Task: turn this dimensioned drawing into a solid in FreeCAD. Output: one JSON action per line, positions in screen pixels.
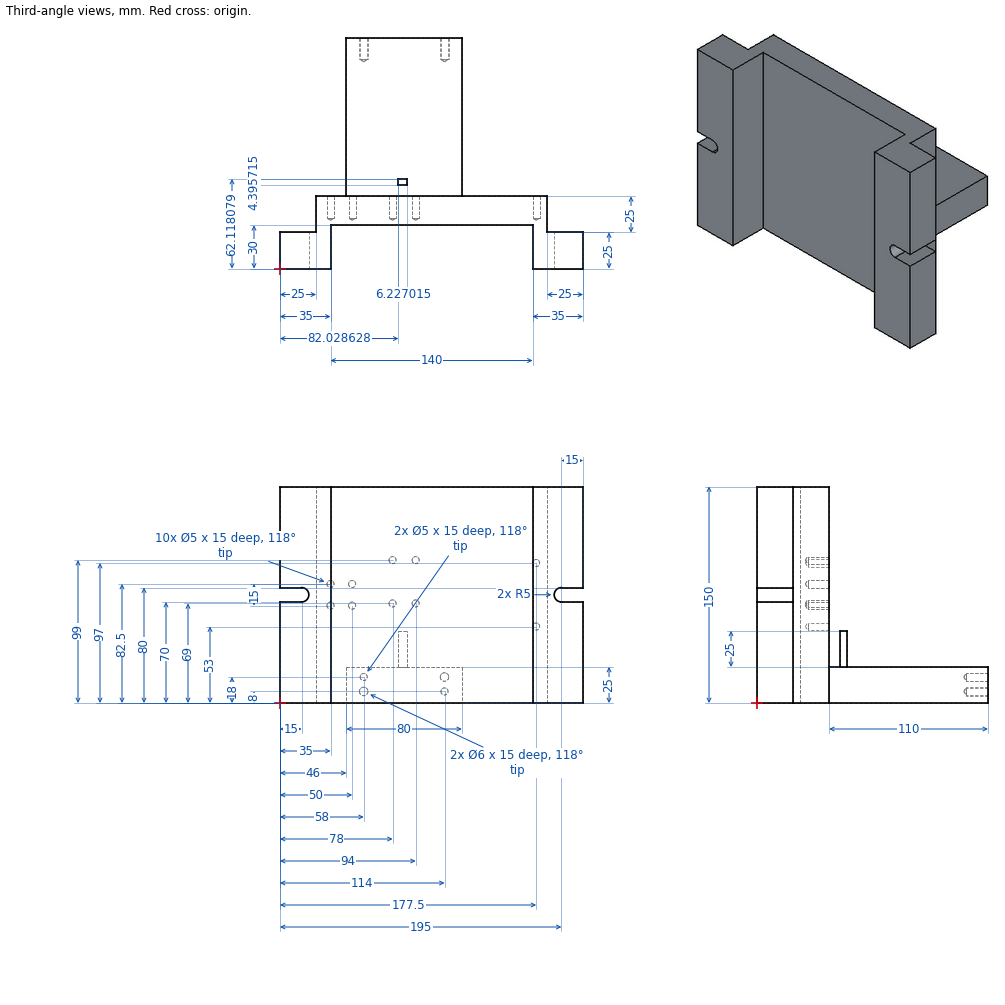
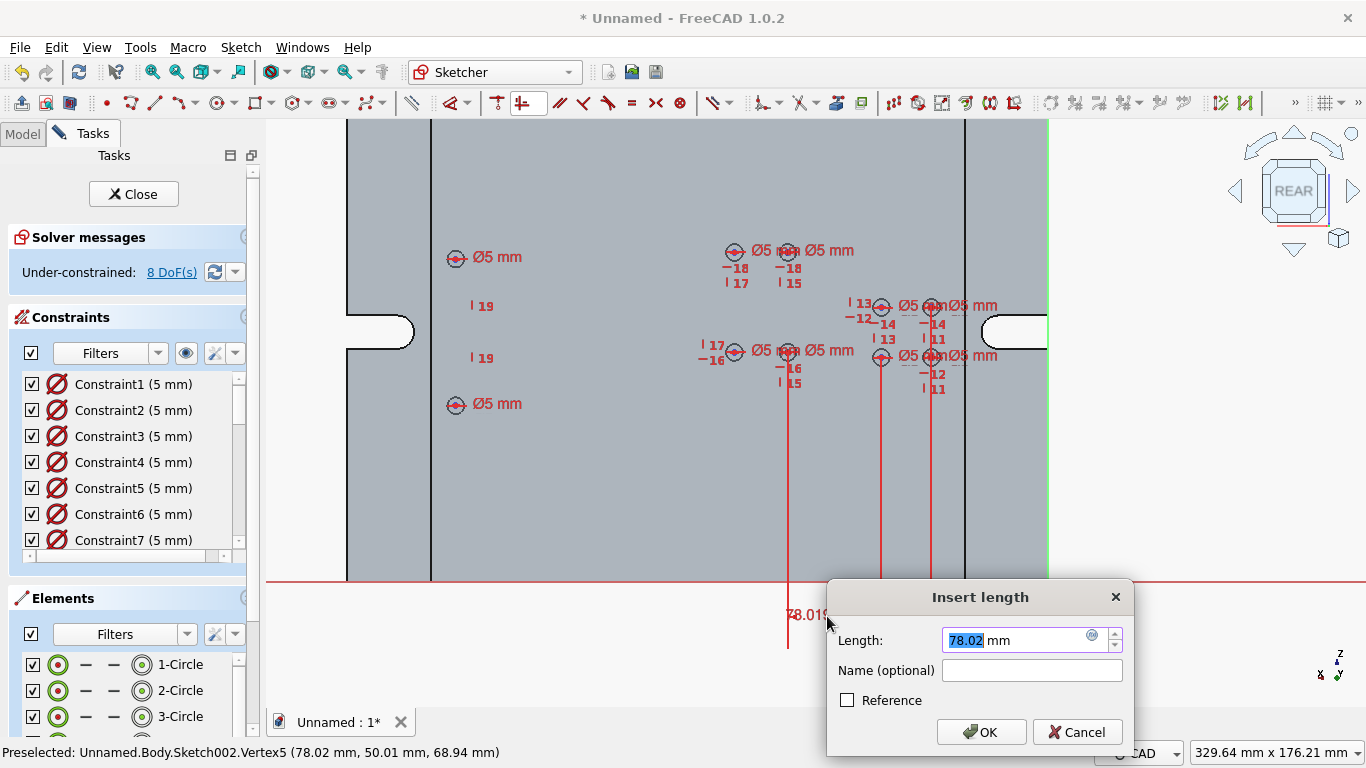
{"action": "type", "text": "78"}
{"action": "key", "text": "Return"}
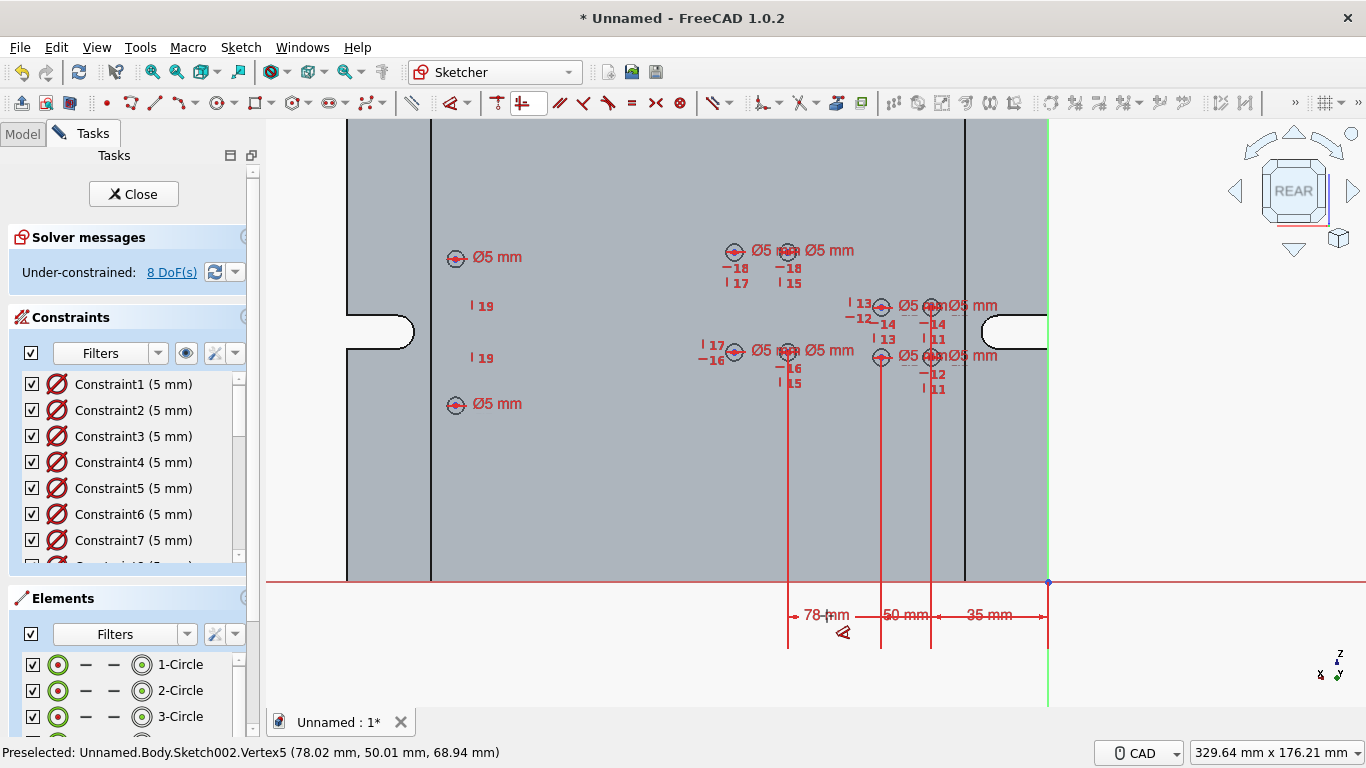
{"action": "left_click", "coordinate": [788, 352]}
{"action": "left_click", "coordinate": [1082, 467]}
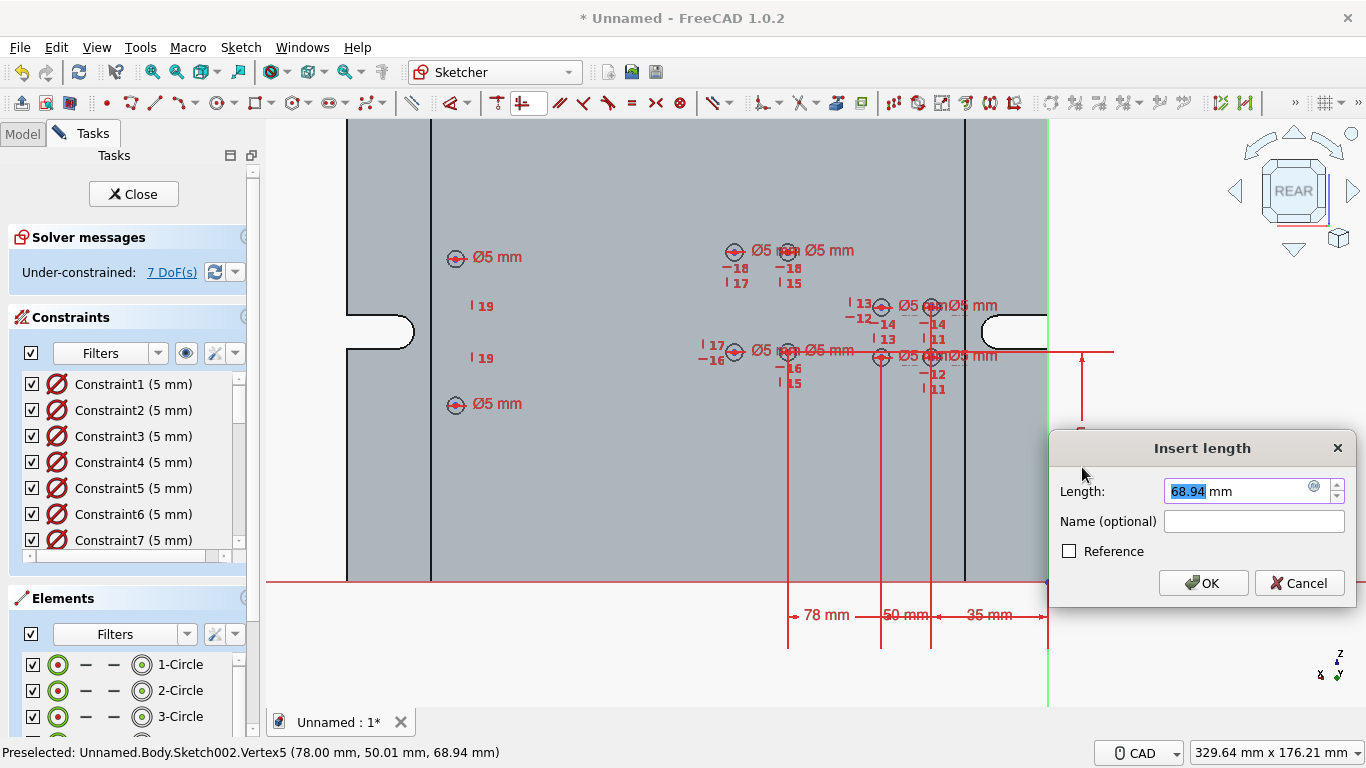
{"action": "type", "text": "69"}
{"action": "key", "text": "Return"}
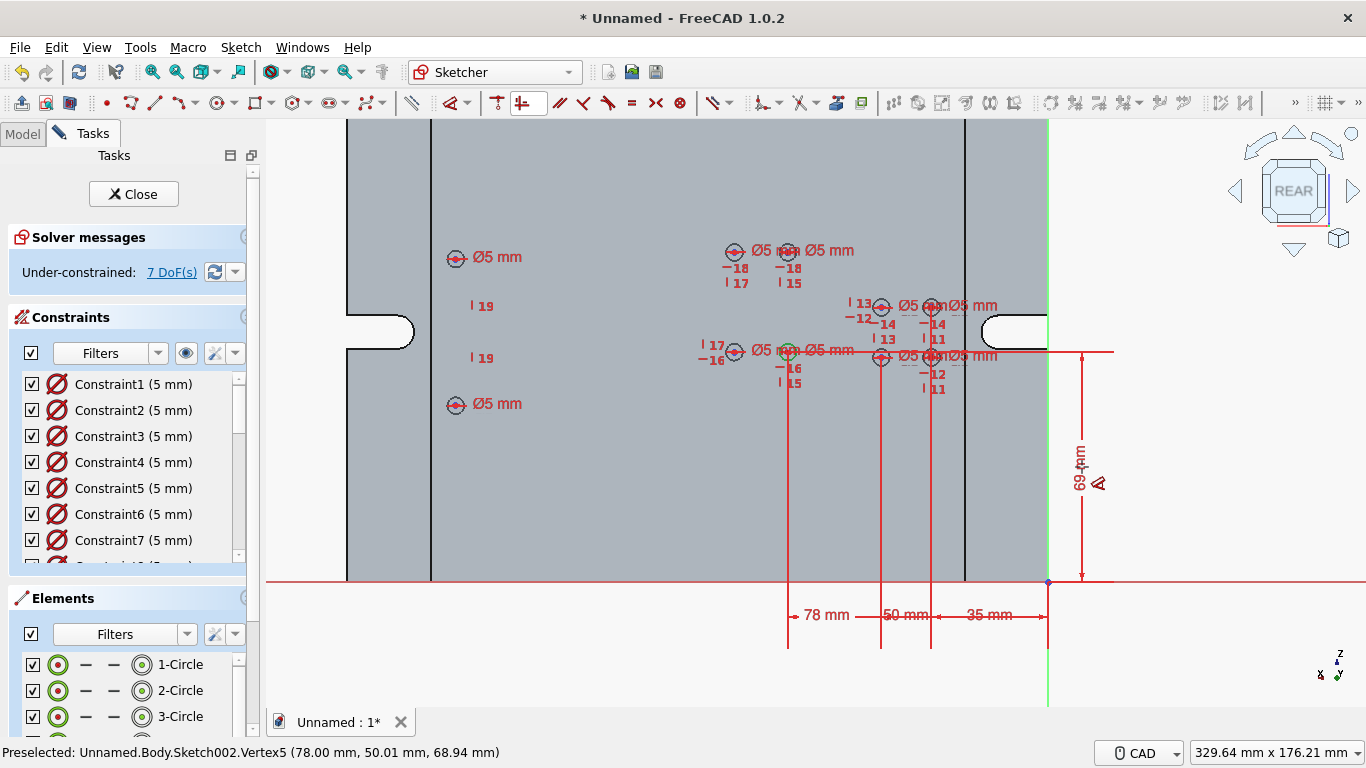
{"action": "left_click", "coordinate": [788, 252]}
{"action": "left_click", "coordinate": [1082, 417]}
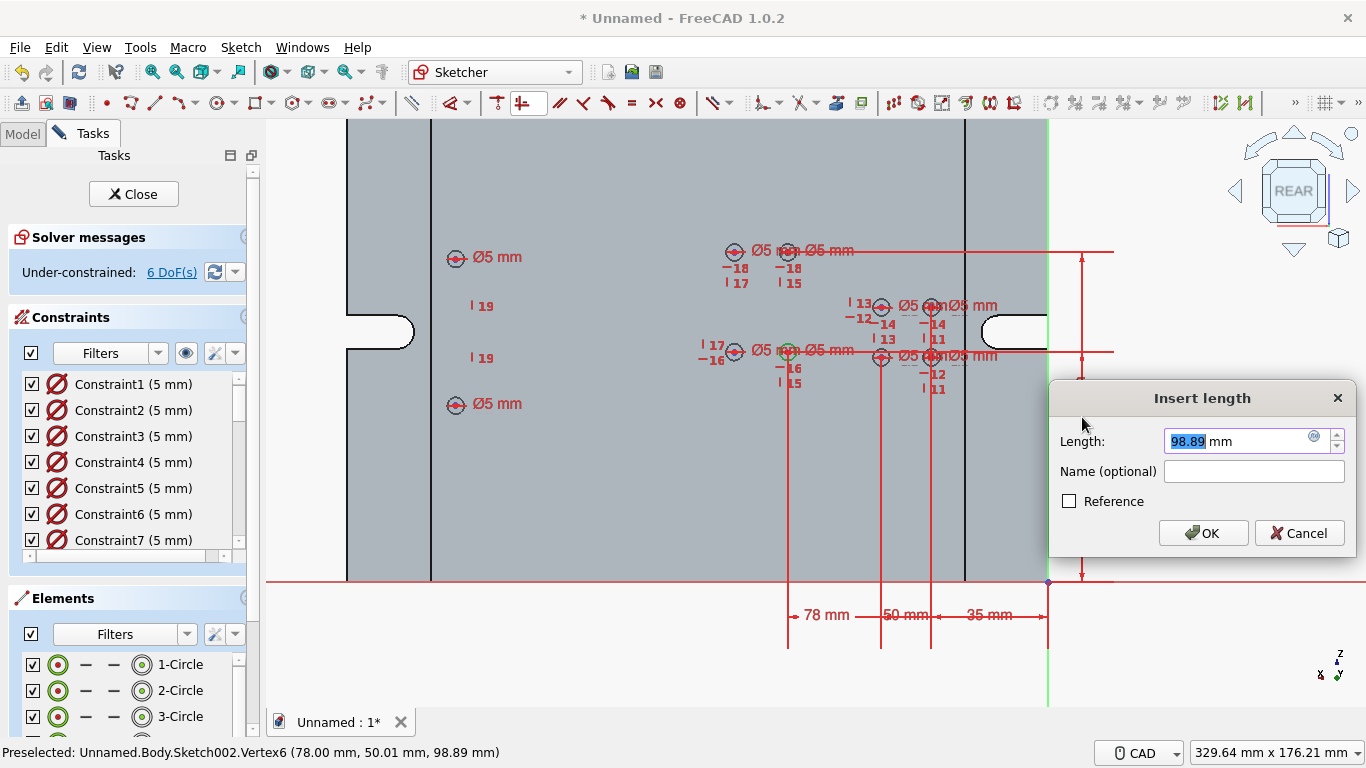
{"action": "type", "text": "99"}
{"action": "key", "text": "Return"}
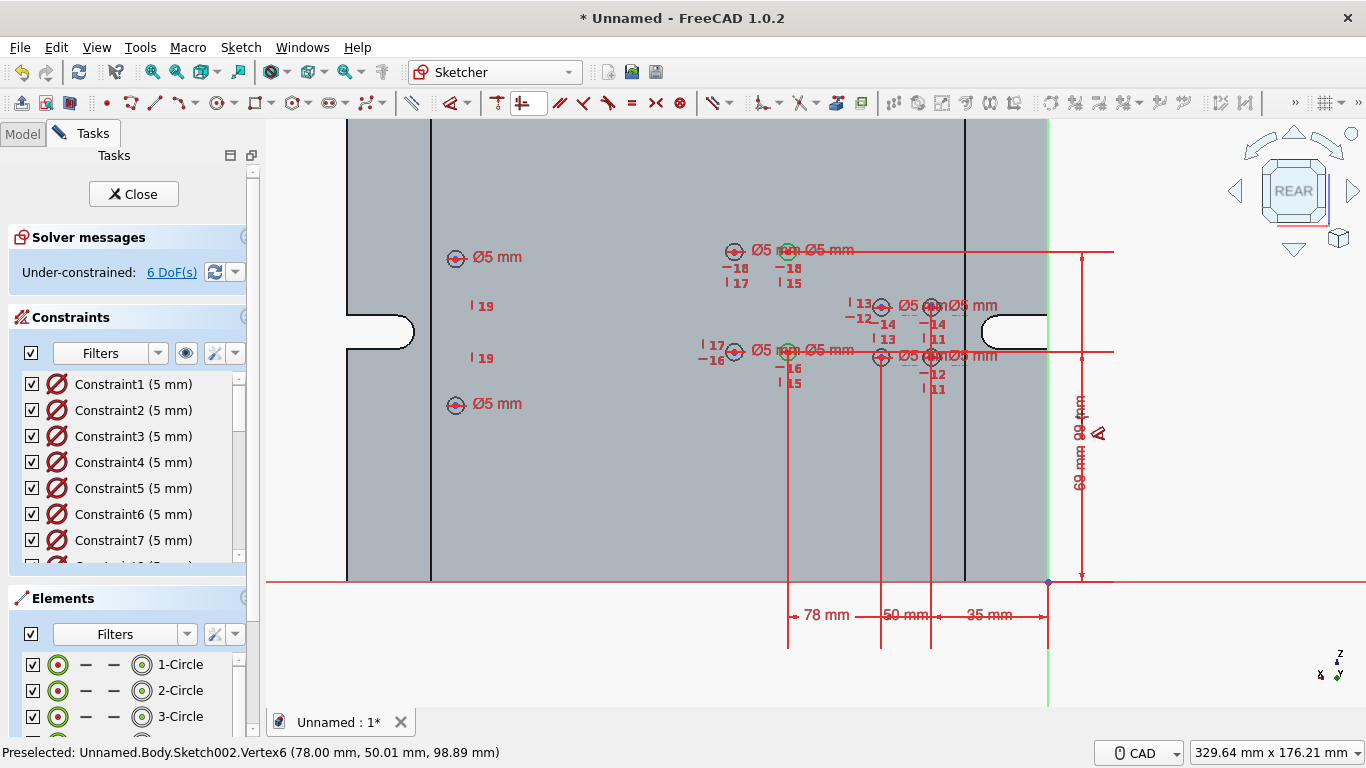
{"action": "left_click", "coordinate": [734, 352]}
{"action": "left_click", "coordinate": [819, 318]}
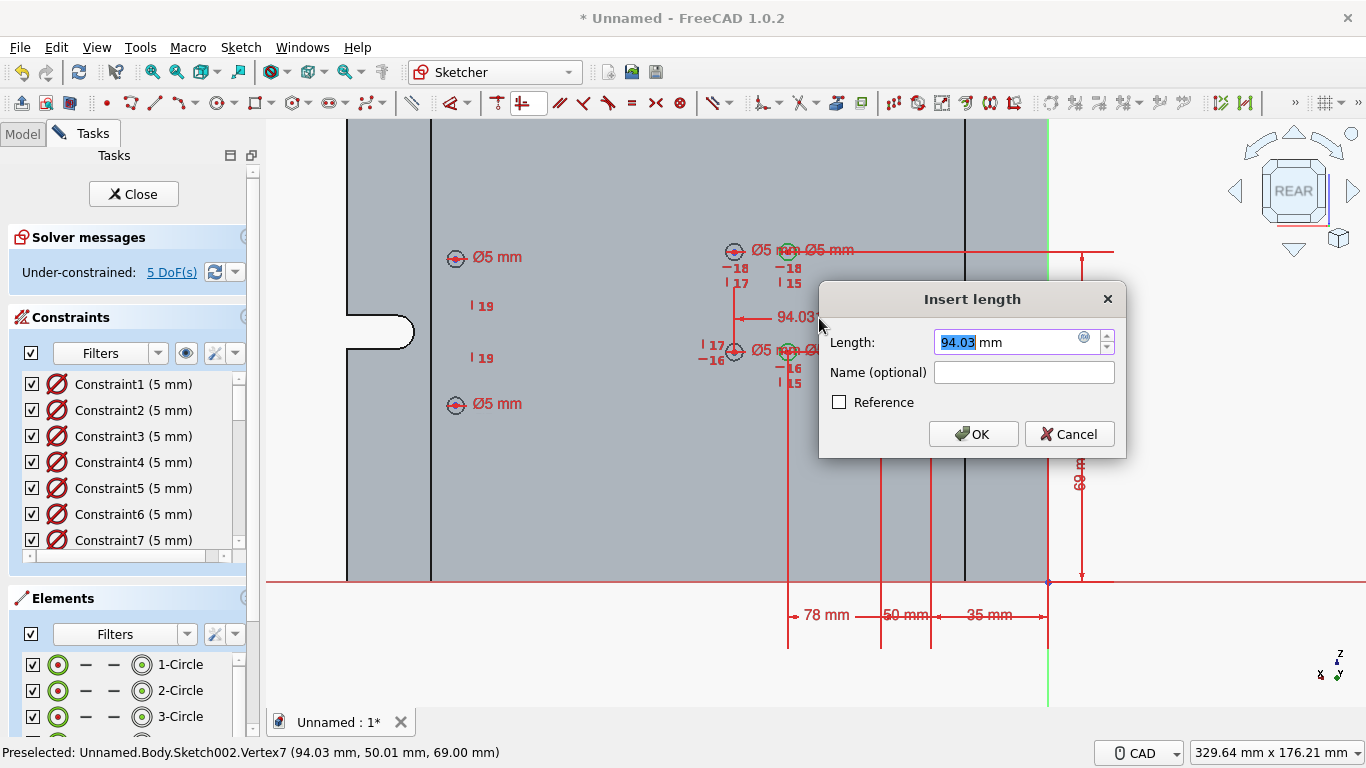
{"action": "type", "text": "94"}
{"action": "key", "text": "Return"}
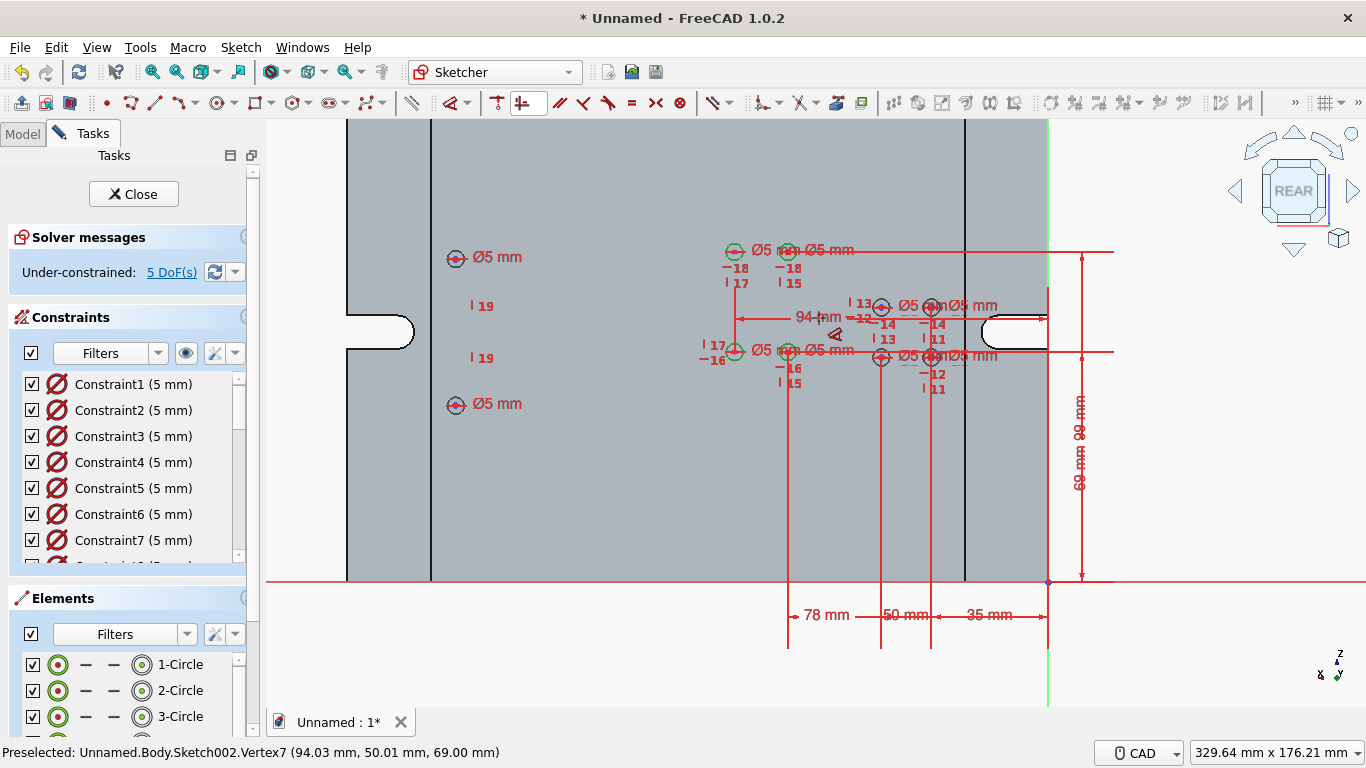
{"action": "left_click", "coordinate": [456, 259]}
{"action": "left_click", "coordinate": [1082, 346]}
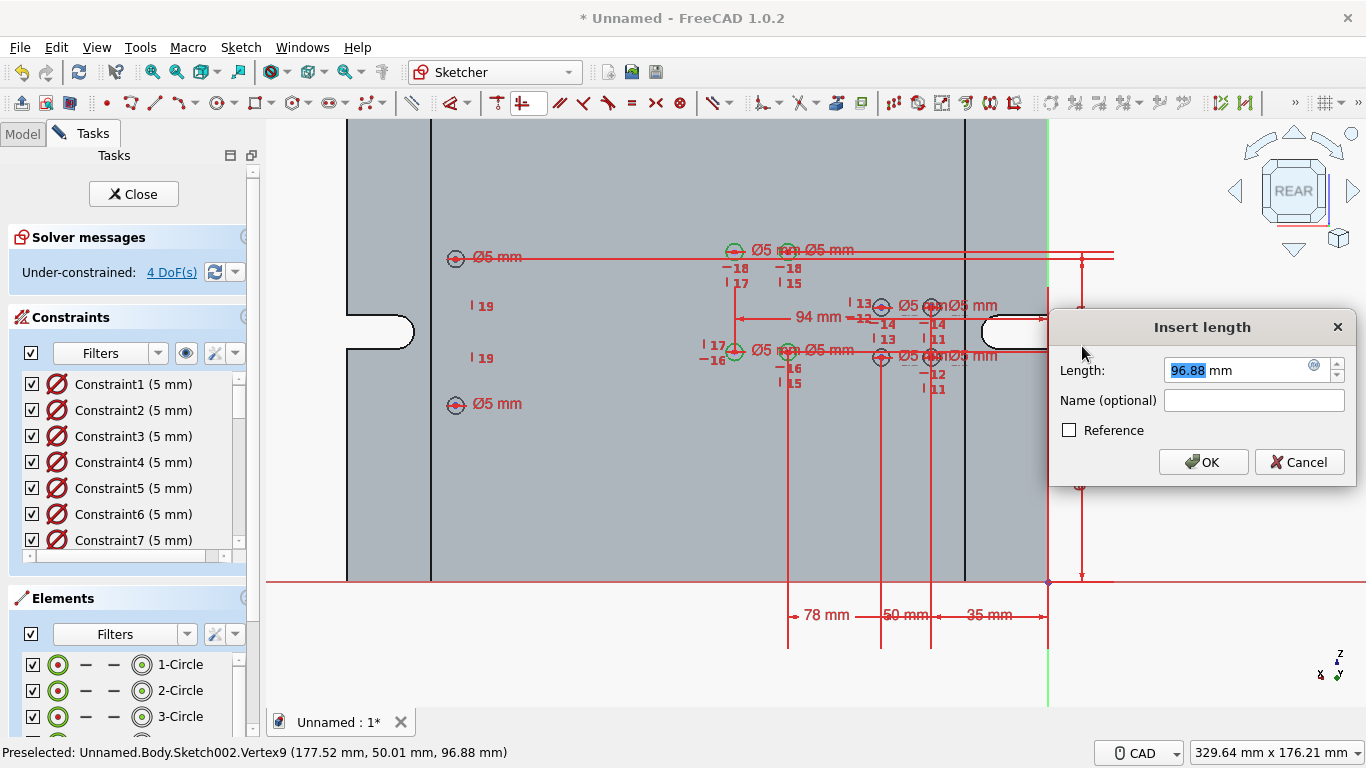
{"action": "type", "text": "97"}
{"action": "key", "text": "Return"}